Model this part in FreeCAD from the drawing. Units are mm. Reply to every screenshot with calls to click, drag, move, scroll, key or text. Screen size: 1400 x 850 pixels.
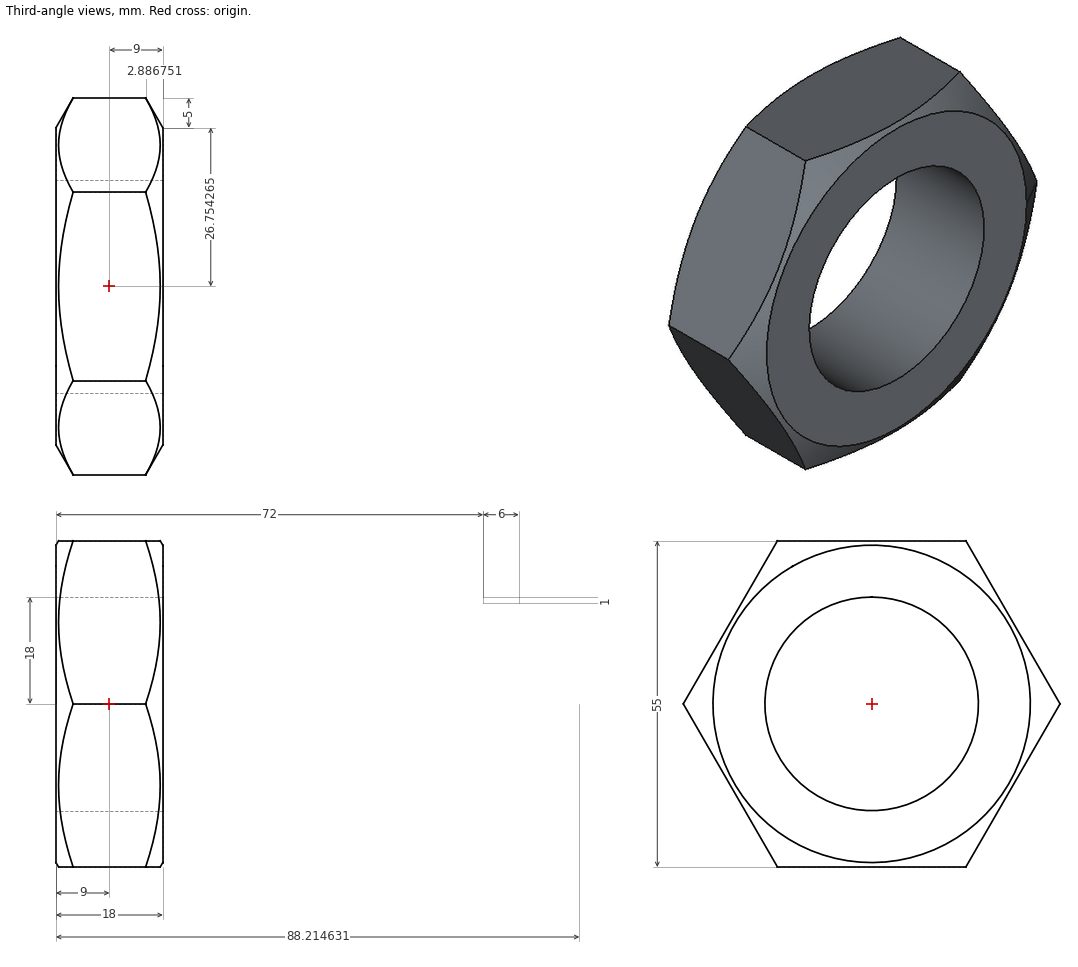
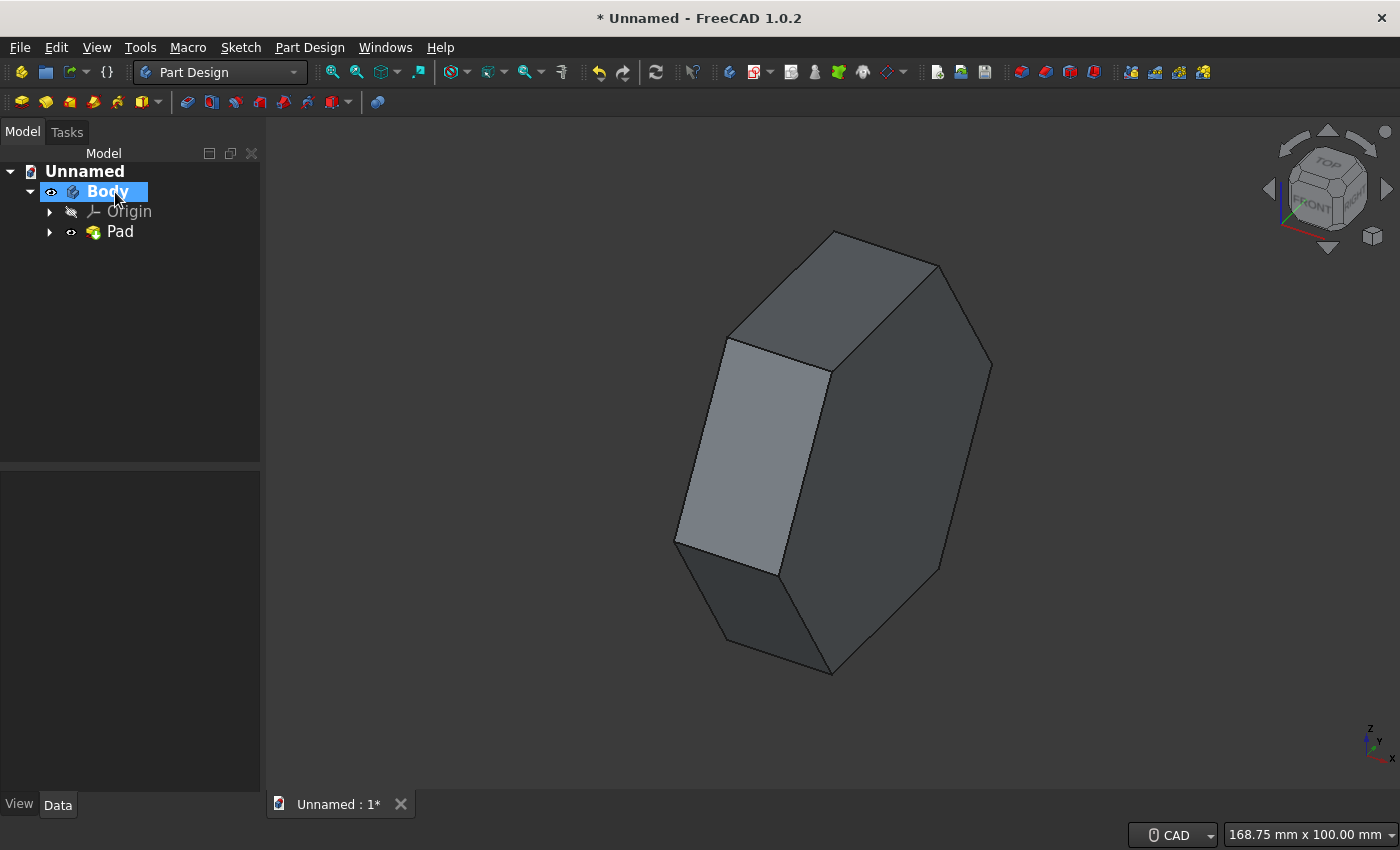
click(754, 72)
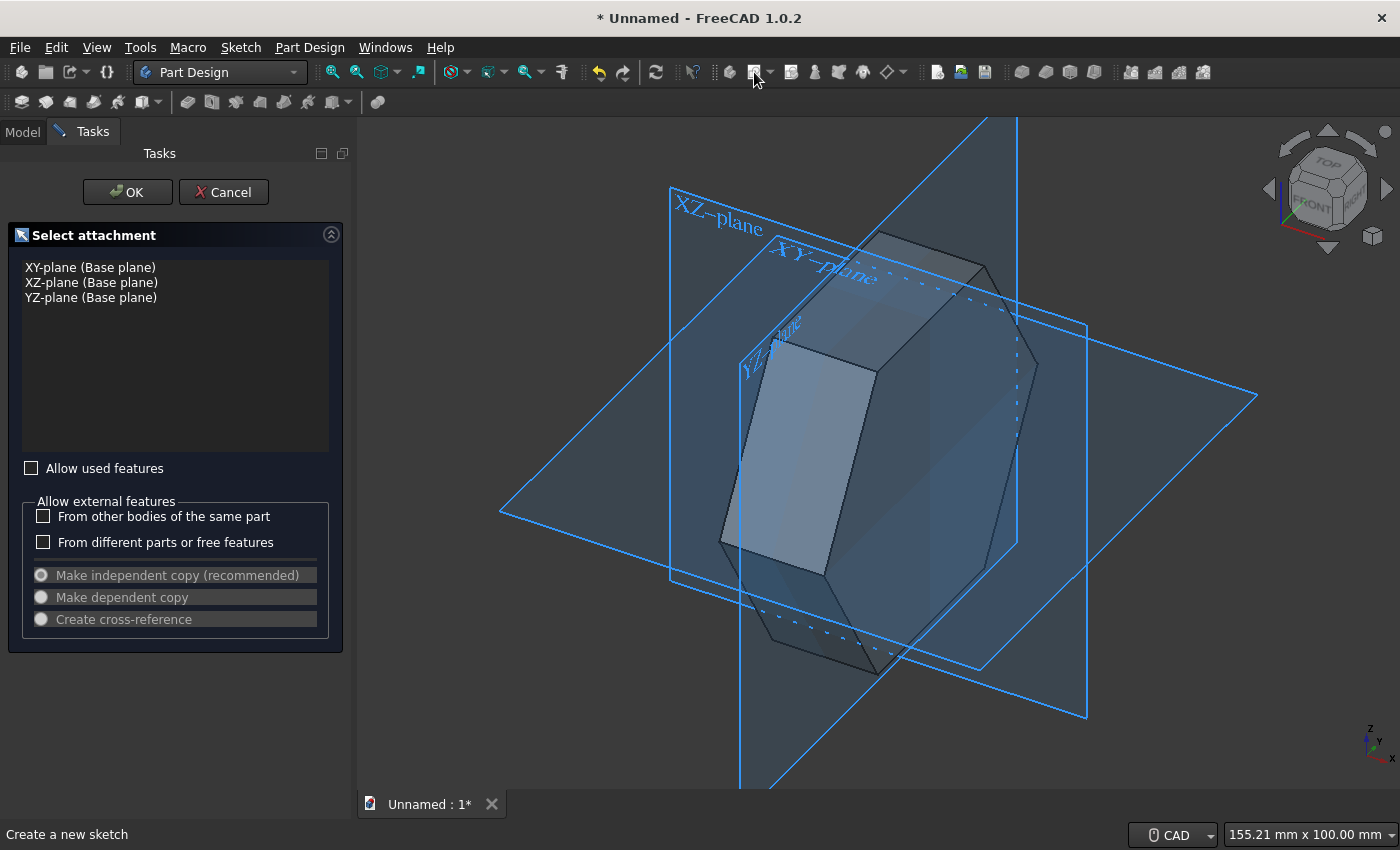
click(82, 282)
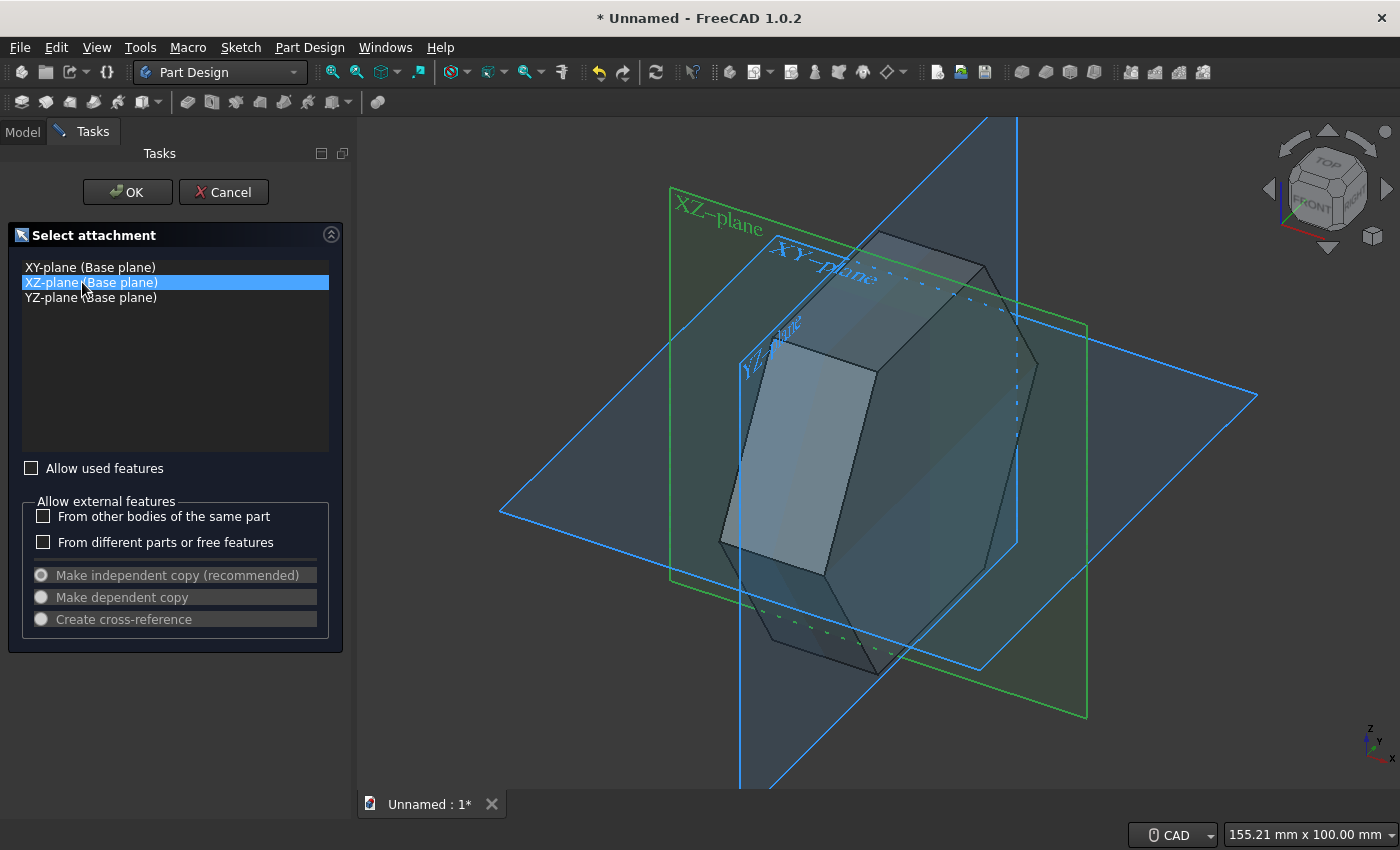
click(128, 192)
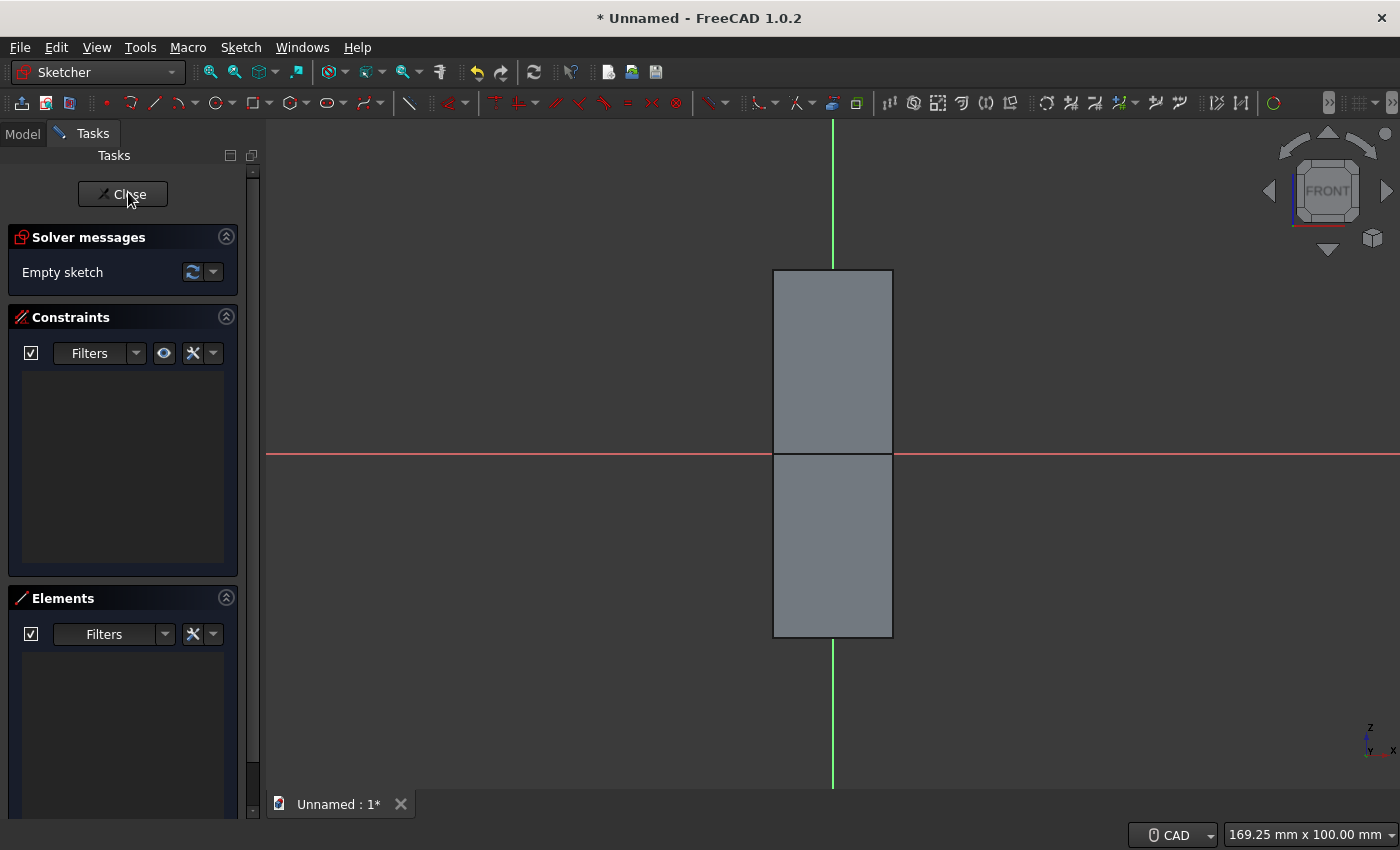
key(q)
key(s)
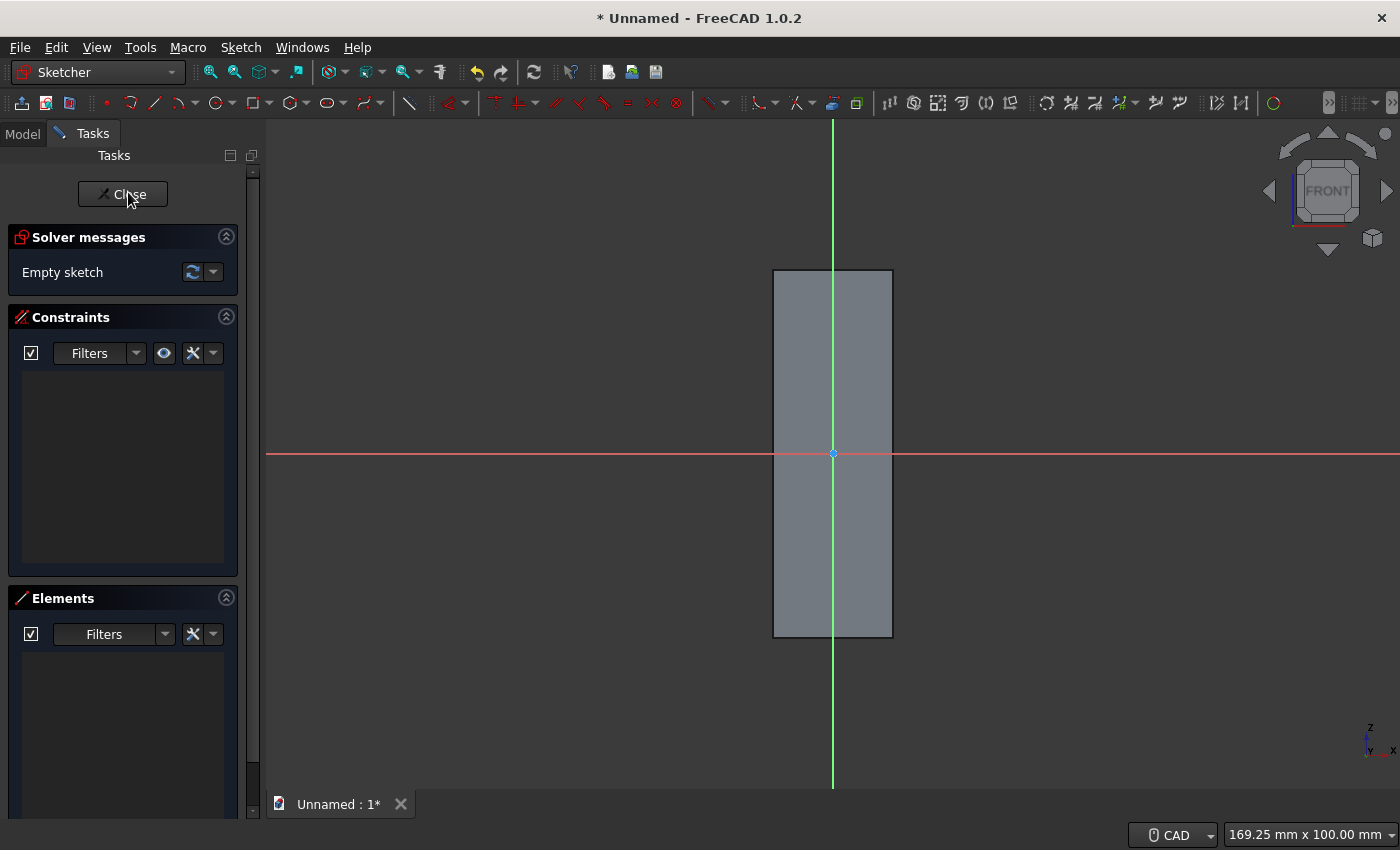
scroll(294, 726, down, 1)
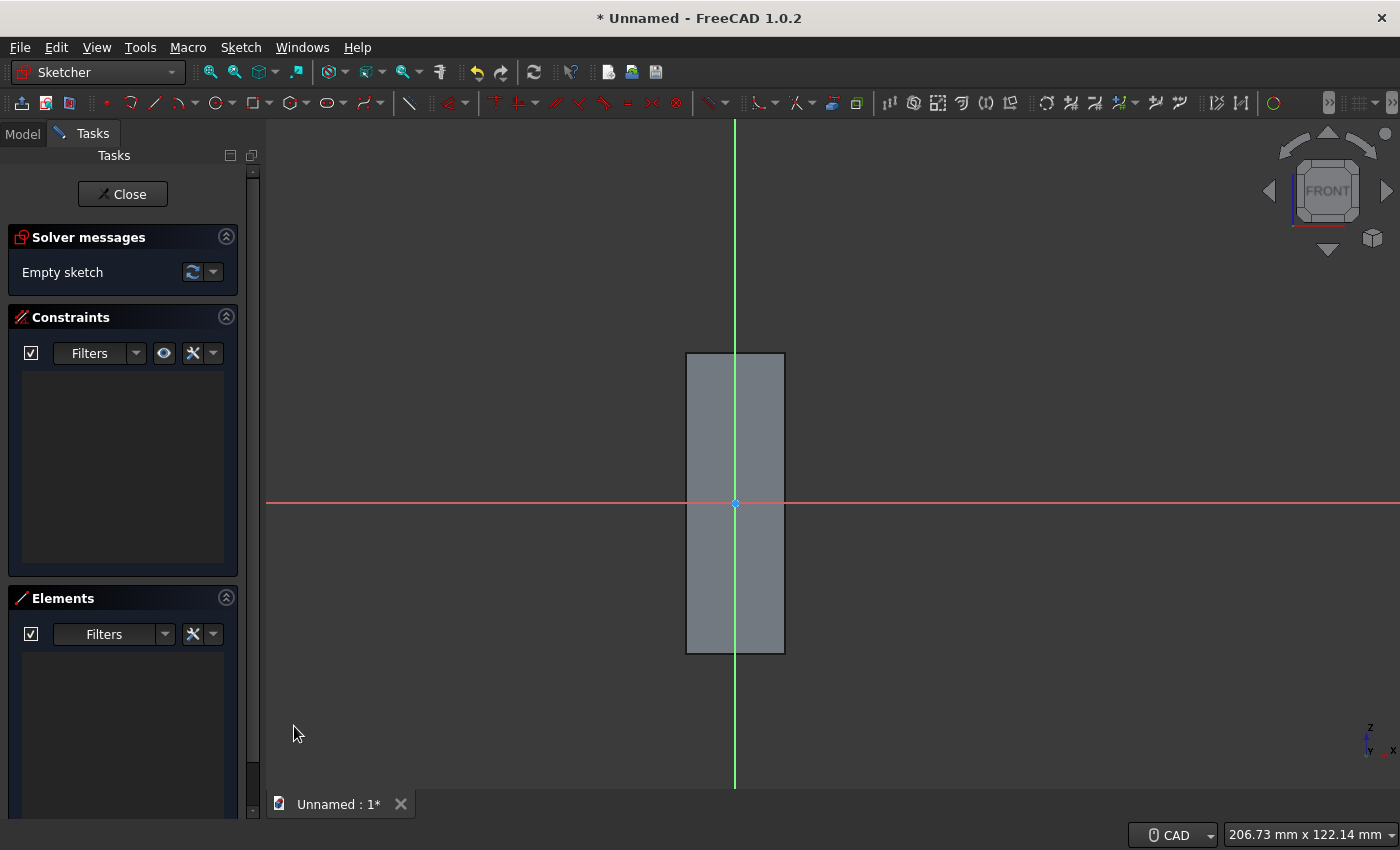
scroll(1235, 454, up, 2)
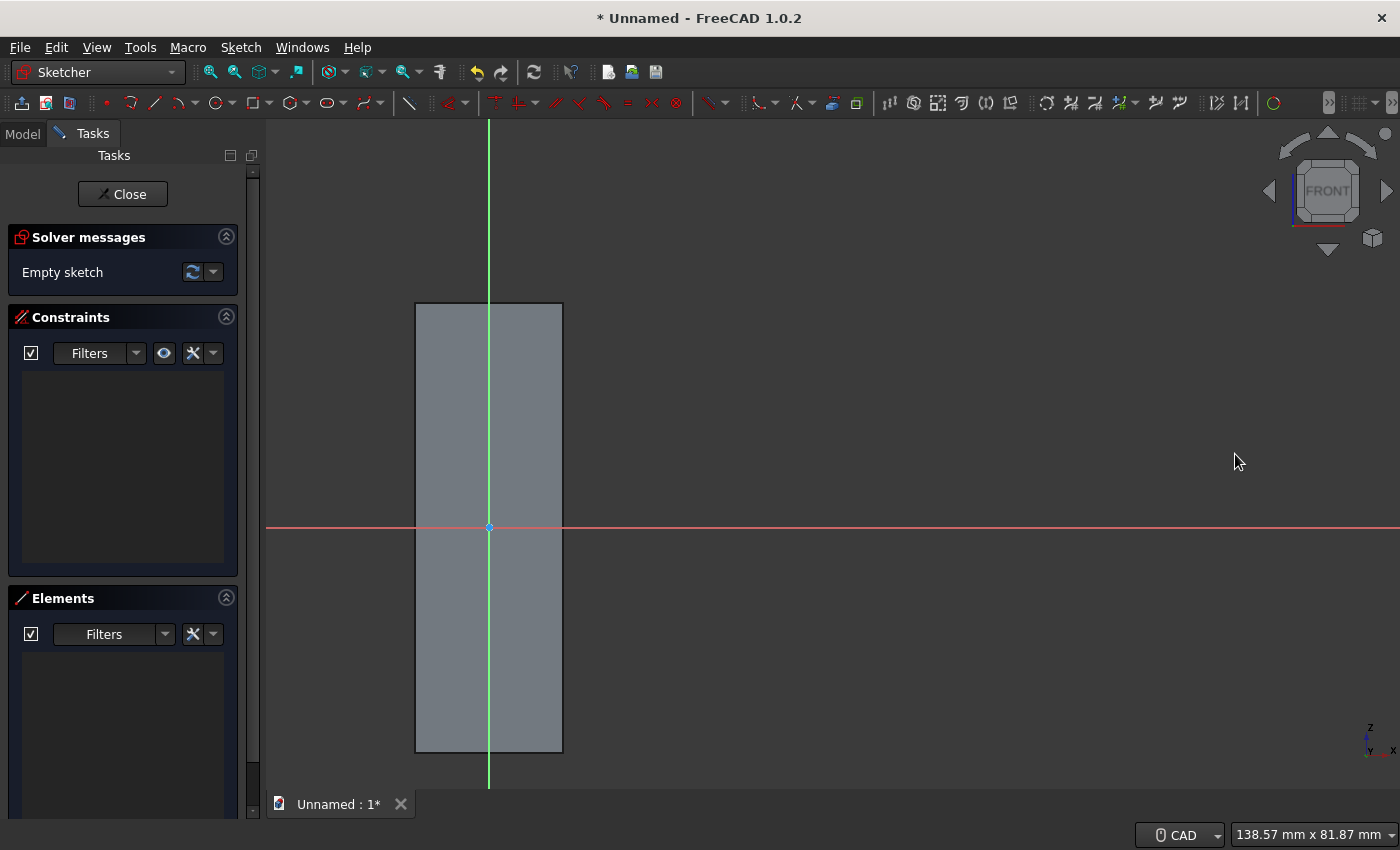
key(g)
key(m)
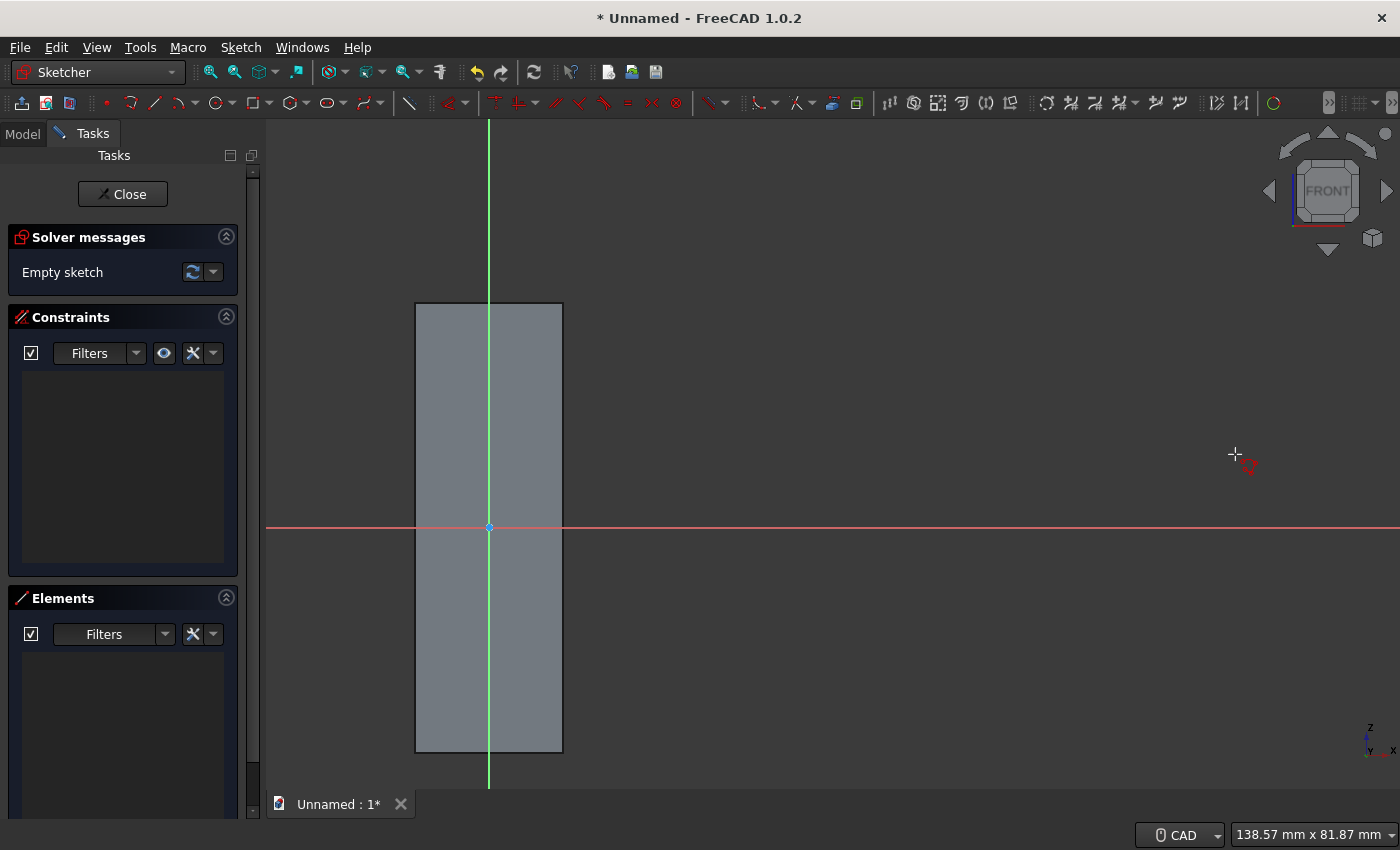
click(415, 528)
click(415, 380)
click(1005, 380)